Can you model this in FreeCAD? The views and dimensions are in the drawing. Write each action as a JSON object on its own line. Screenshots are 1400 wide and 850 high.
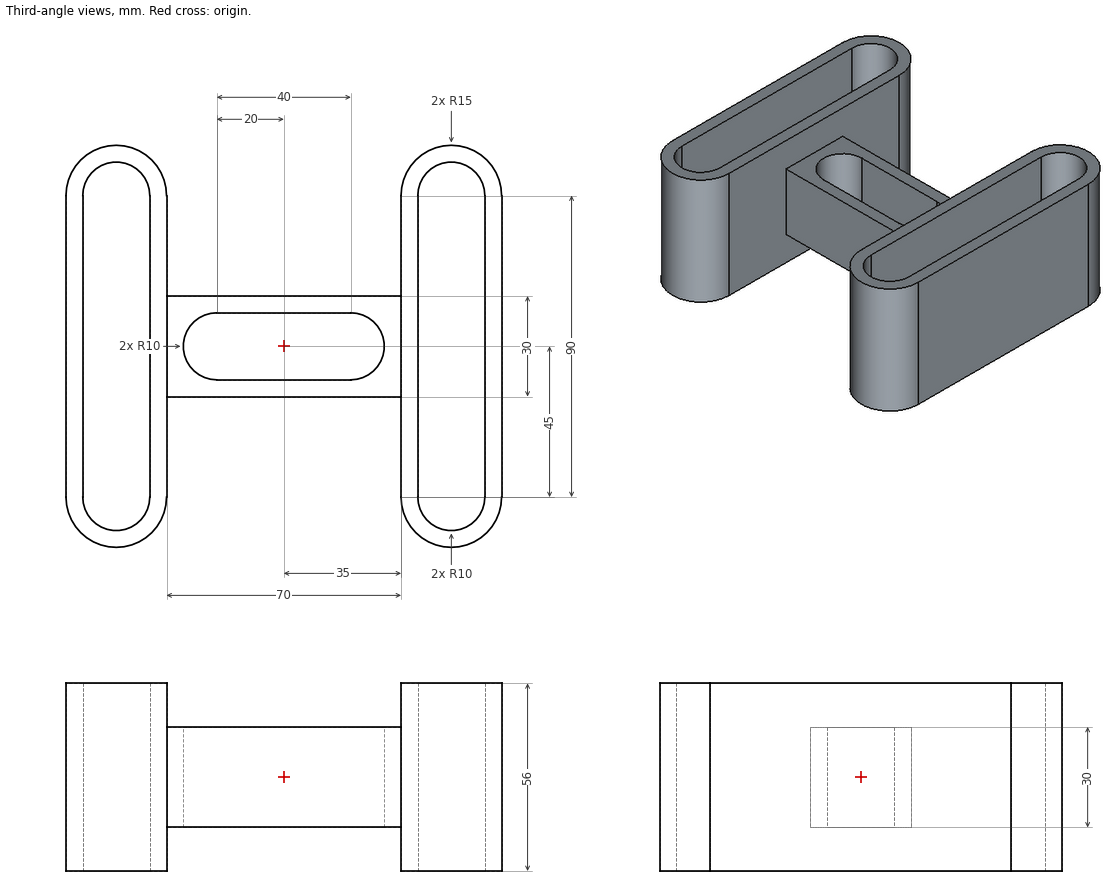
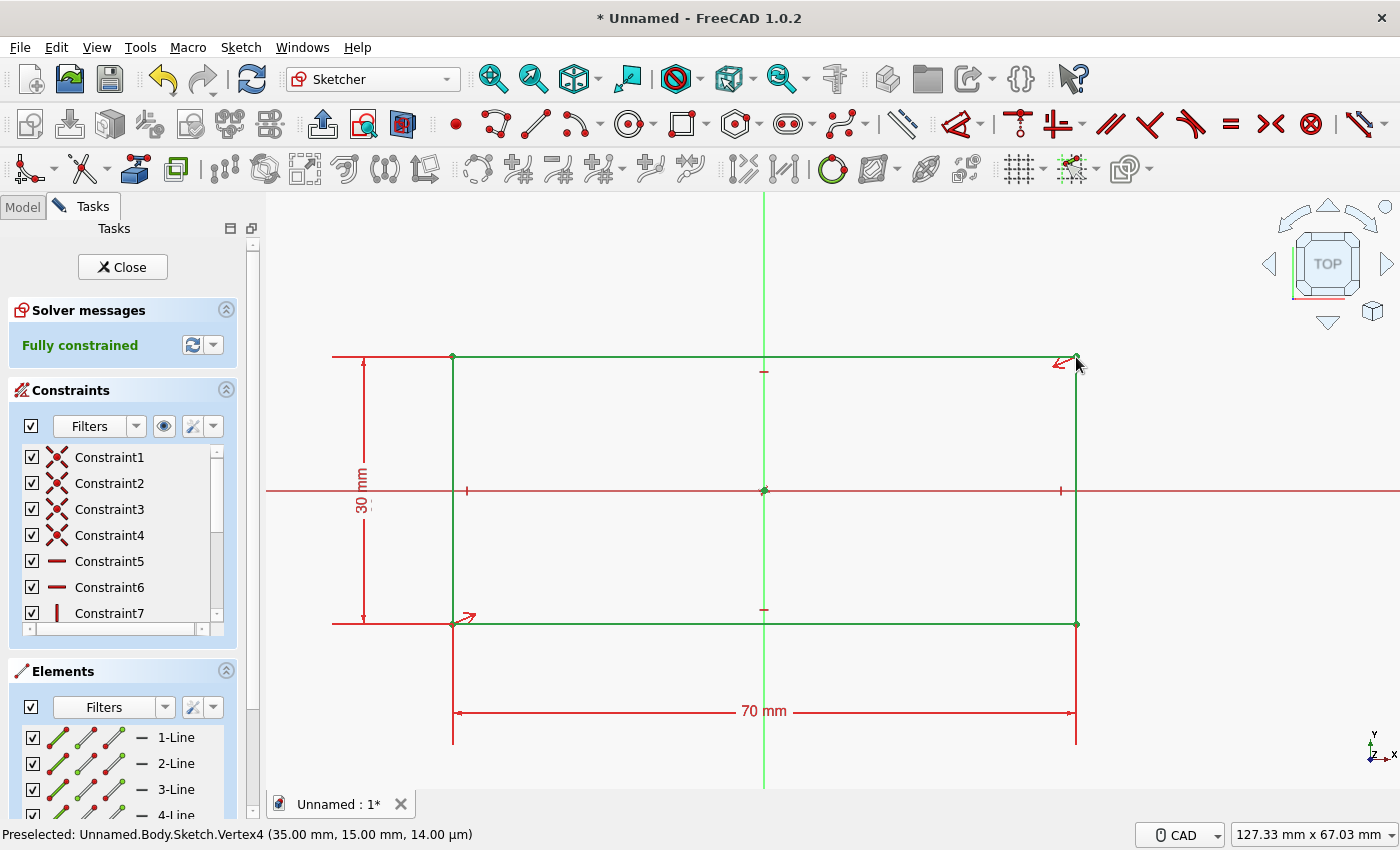
{"action": "left_click", "coordinate": [123, 267]}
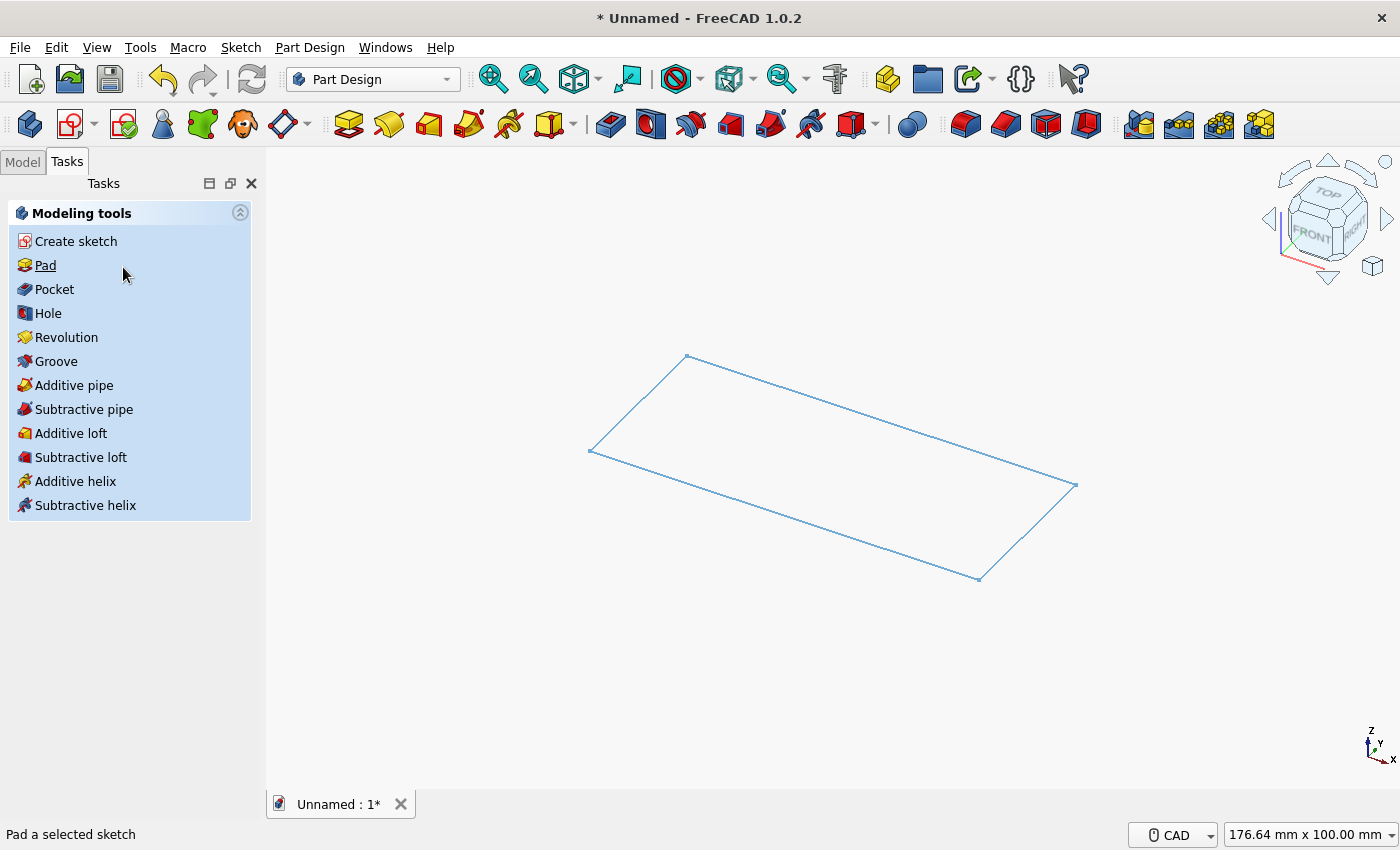
{"action": "left_click", "coordinate": [350, 124]}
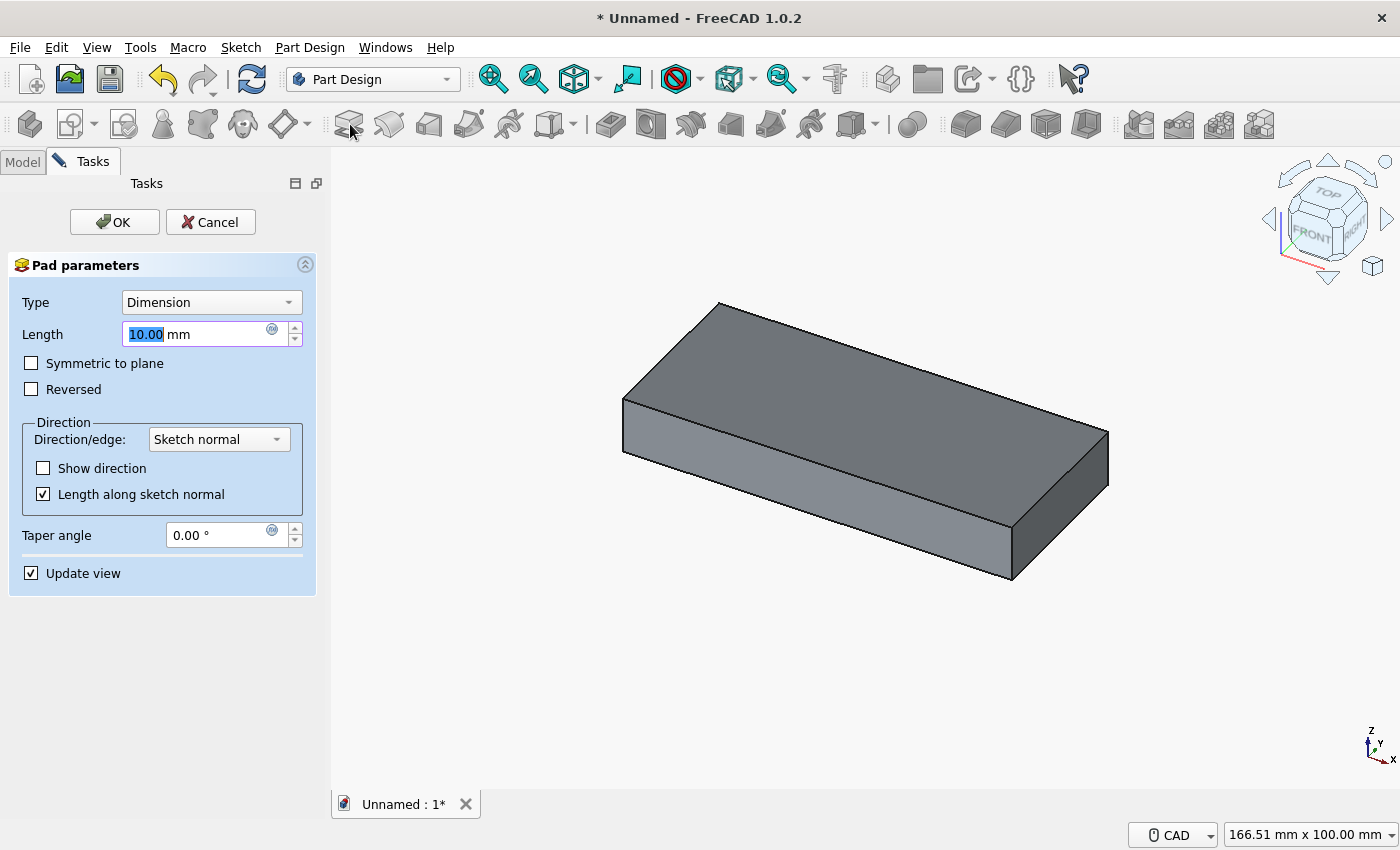
{"action": "type", "text": "30"}
{"action": "key", "text": "Tab"}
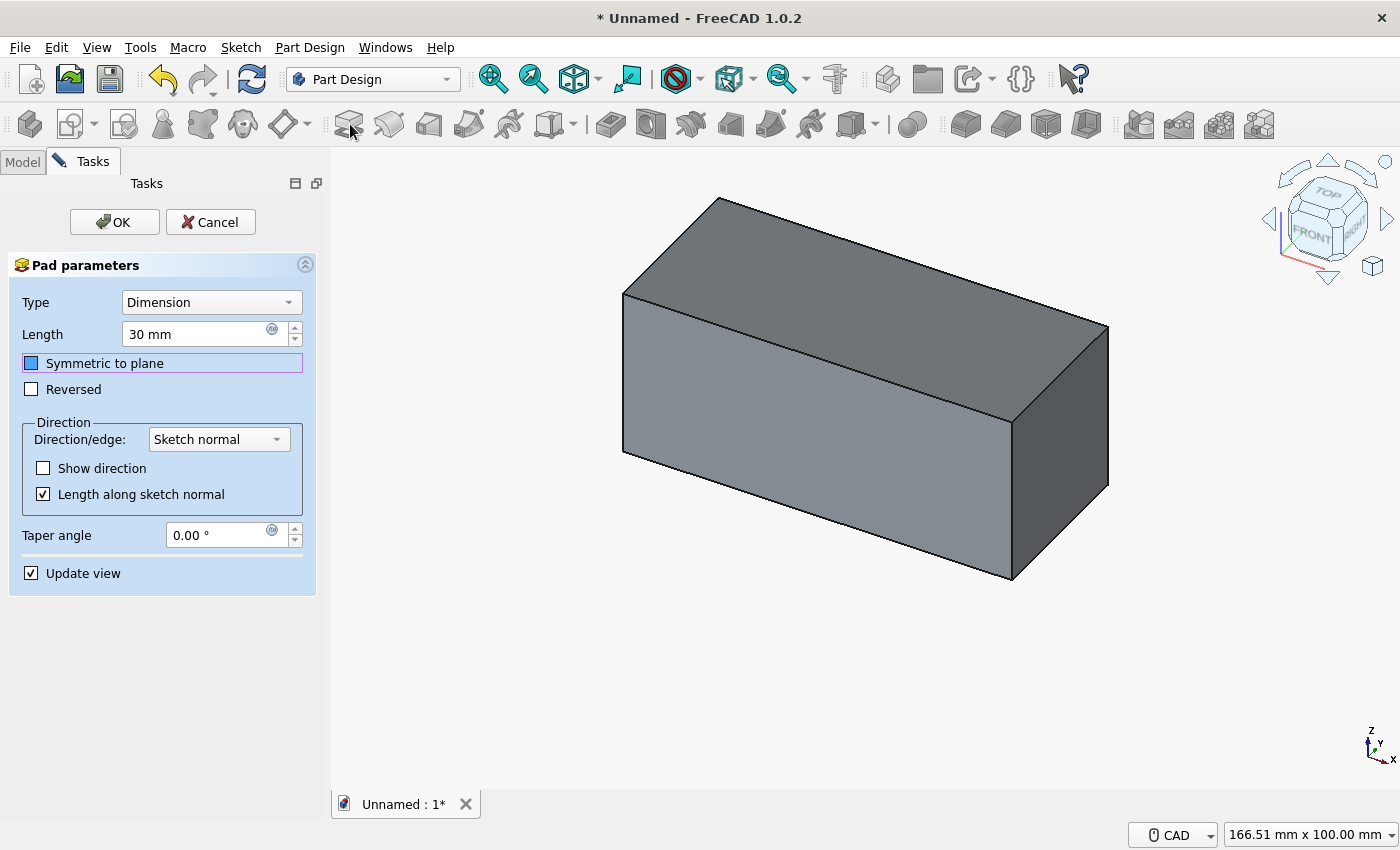
{"action": "left_click", "coordinate": [30, 363]}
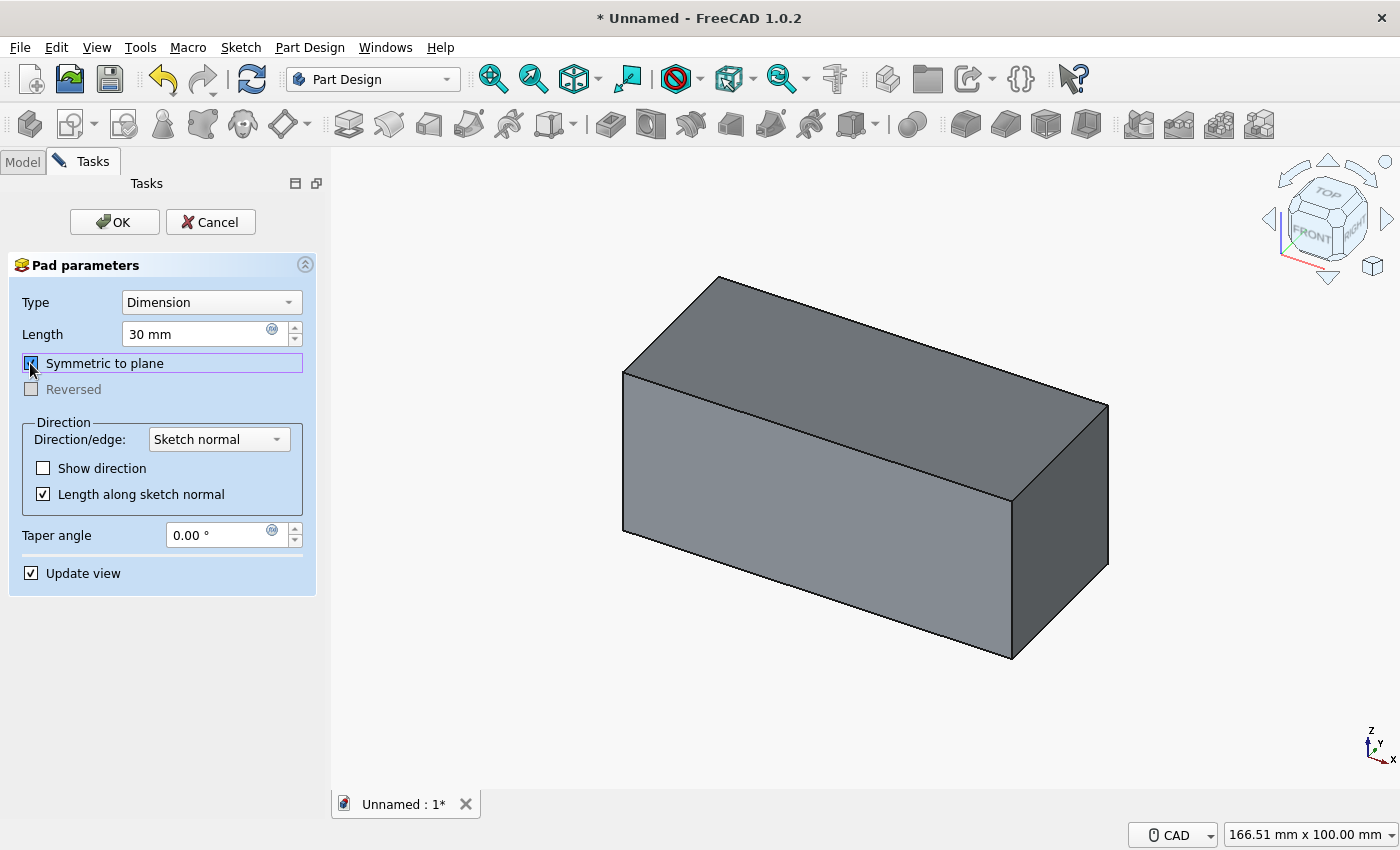
{"action": "left_click", "coordinate": [115, 222]}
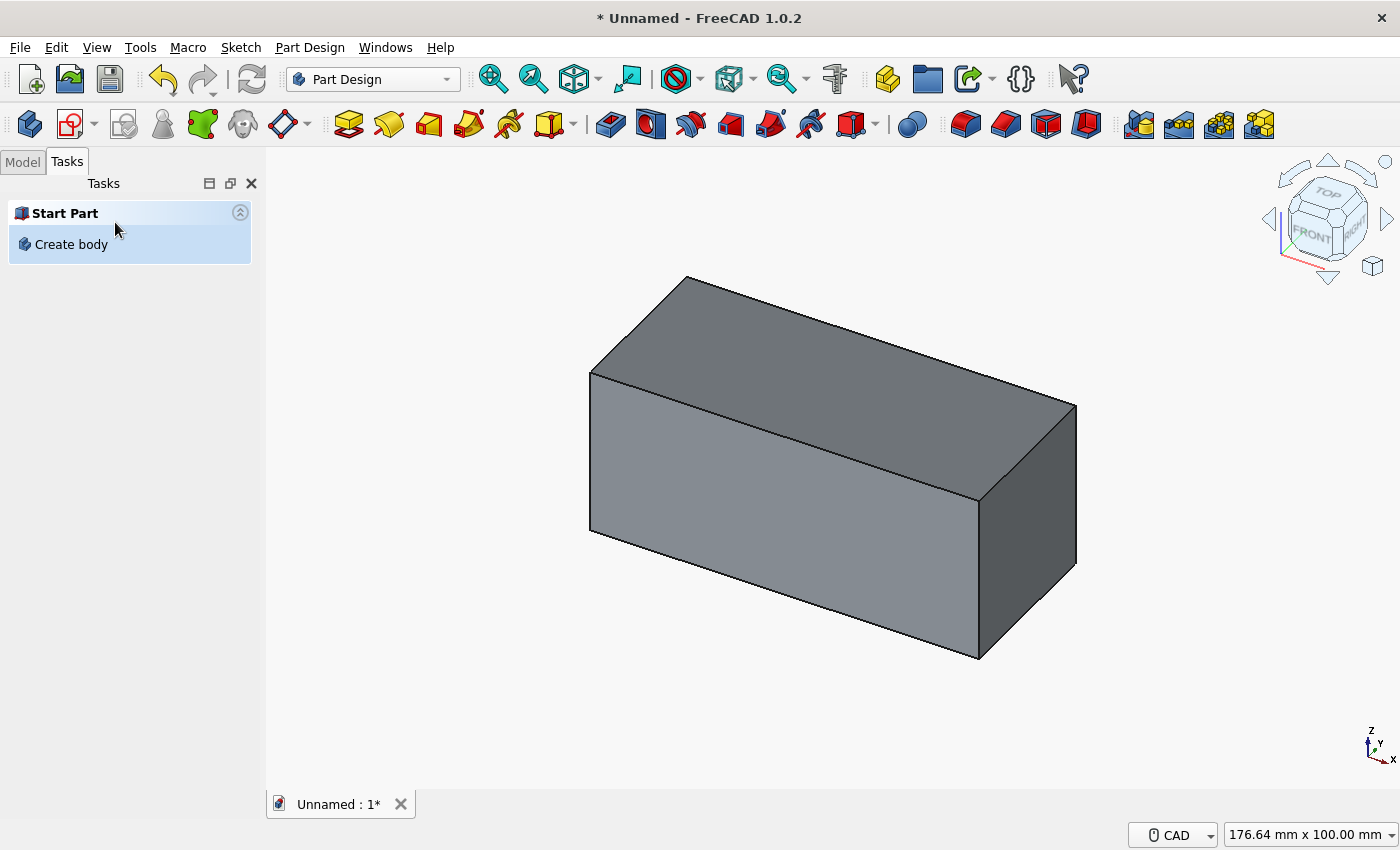
{"action": "left_click", "coordinate": [944, 425]}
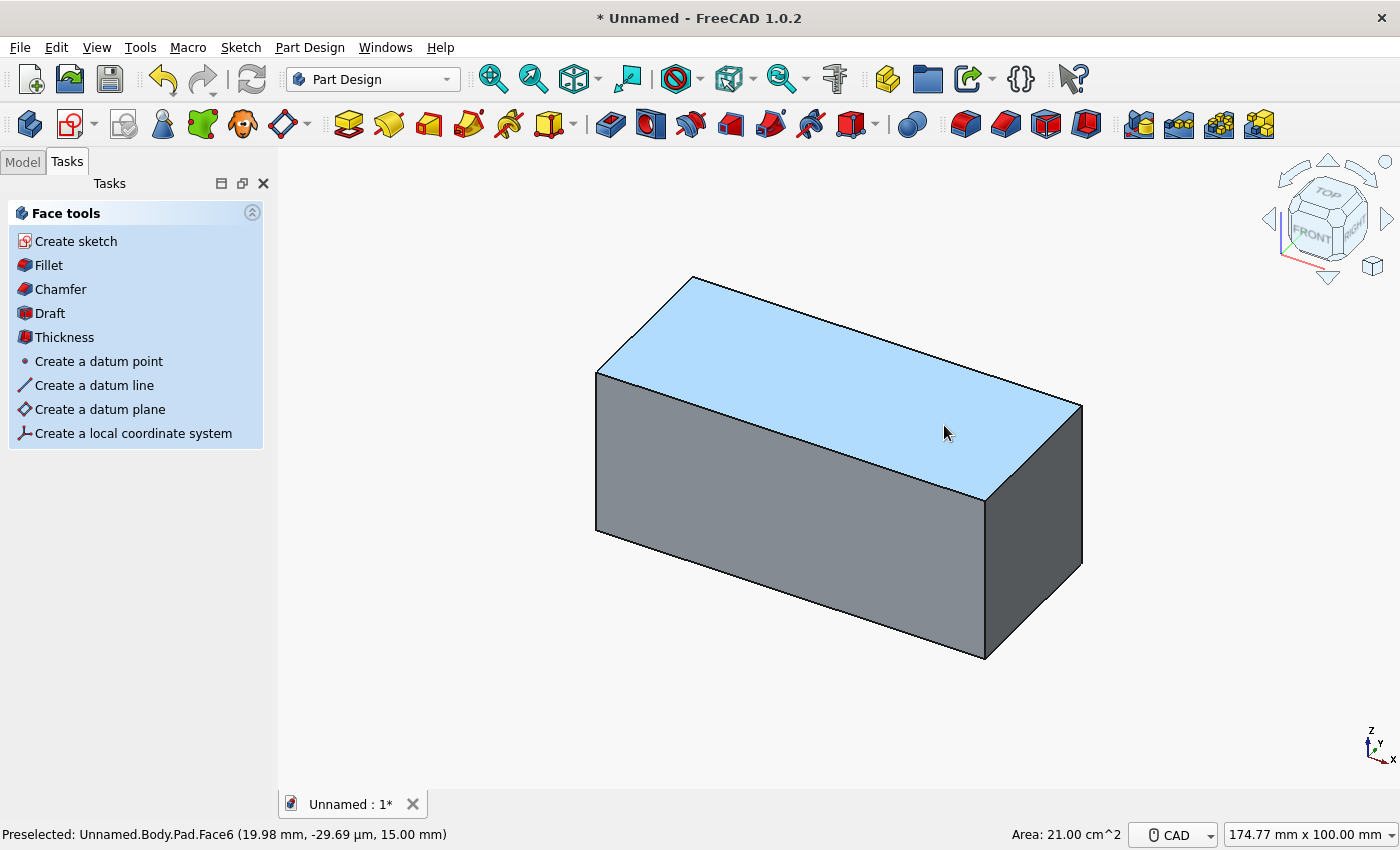
{"action": "left_click", "coordinate": [70, 124]}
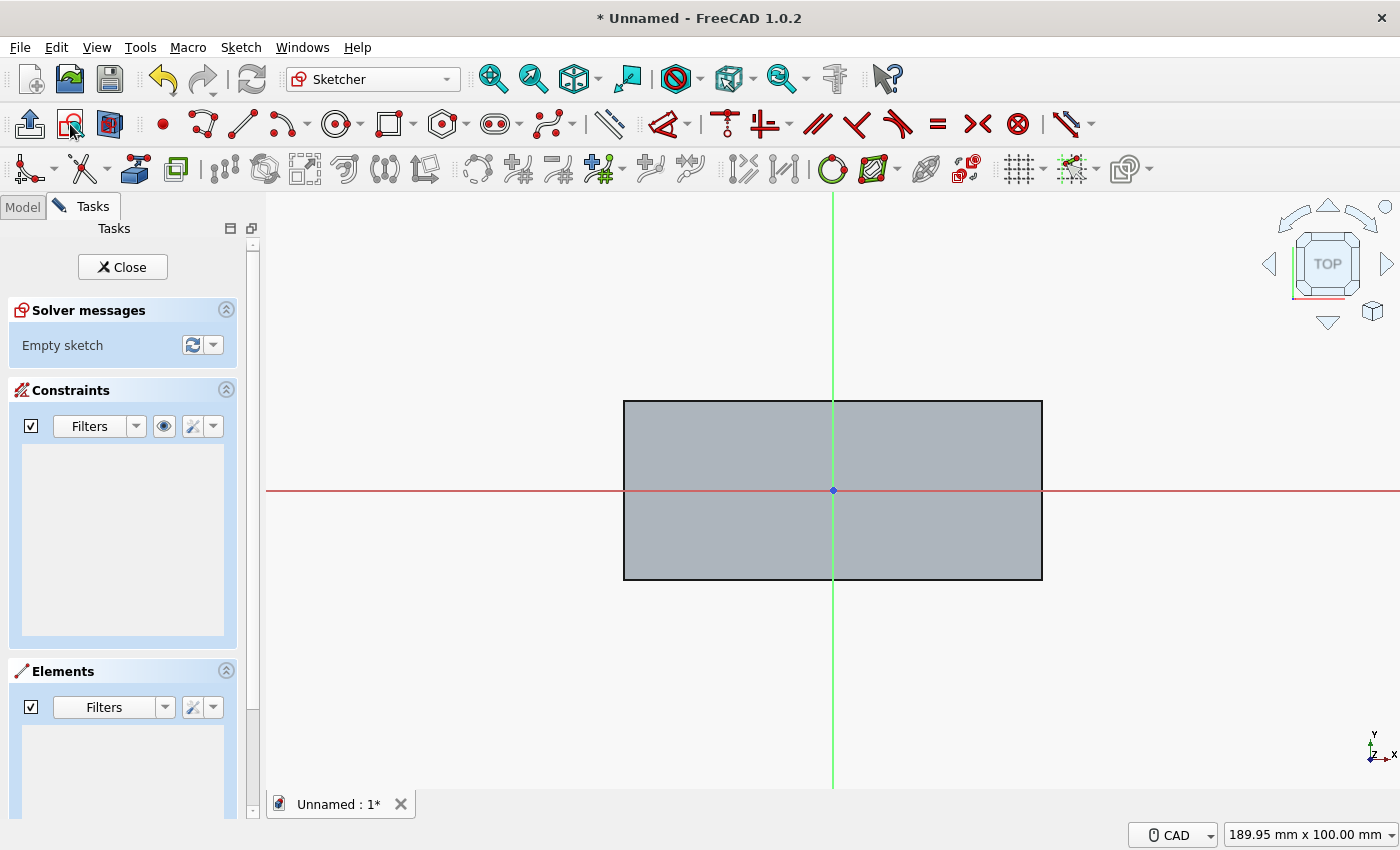
{"action": "scroll", "coordinate": [916, 490], "scroll_direction": "up", "scroll_amount": 3}